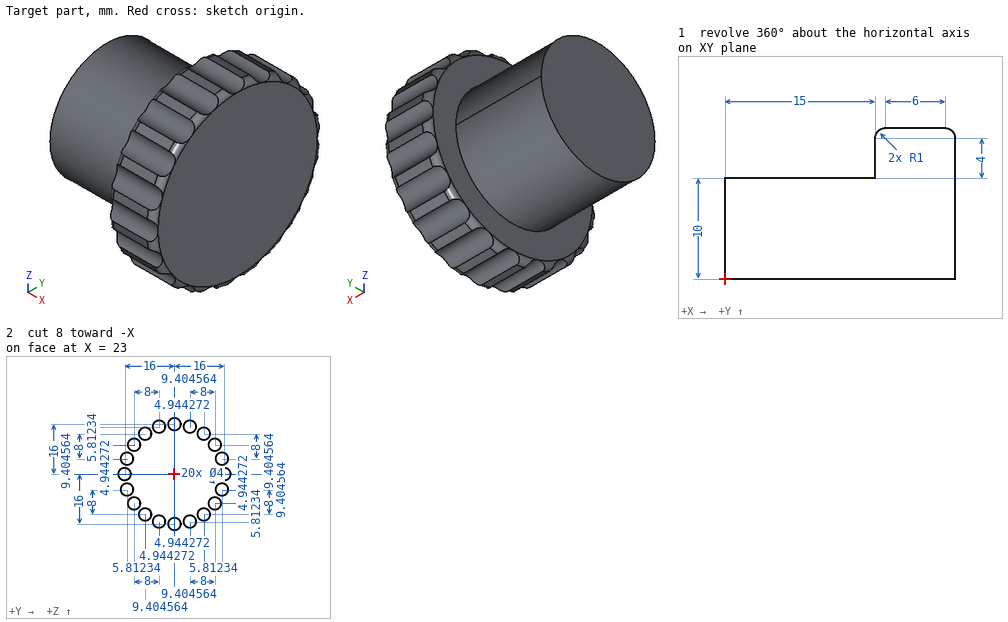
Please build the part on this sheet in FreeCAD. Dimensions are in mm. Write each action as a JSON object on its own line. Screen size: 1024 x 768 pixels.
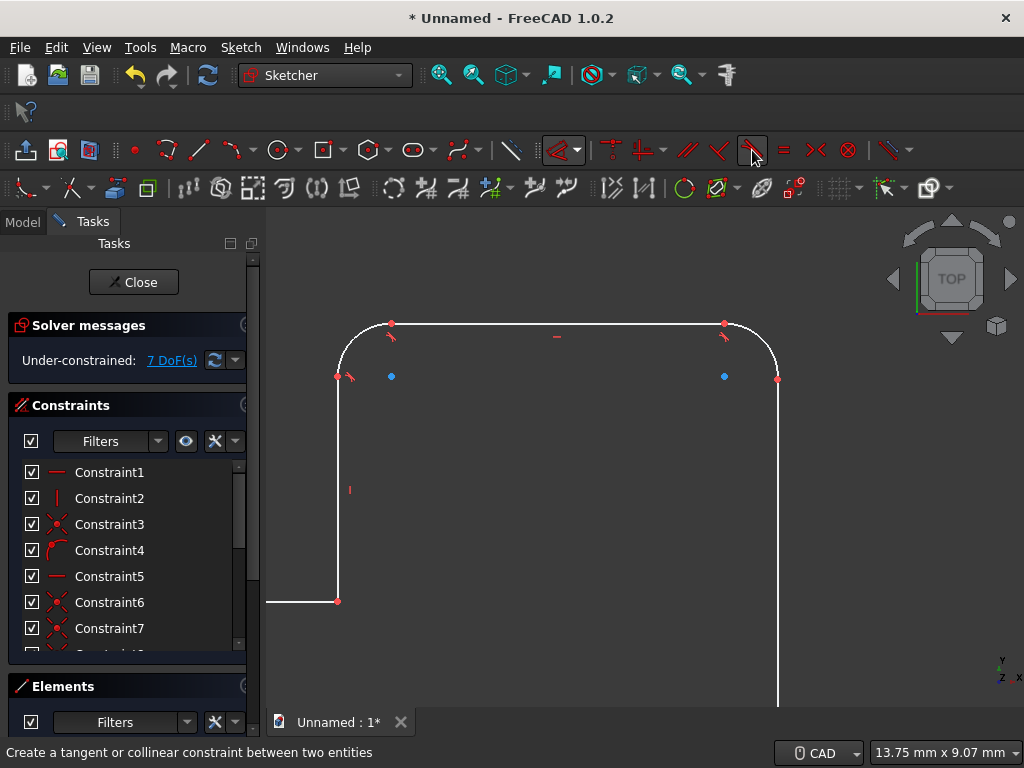
{"action": "left_click", "coordinate": [778, 611]}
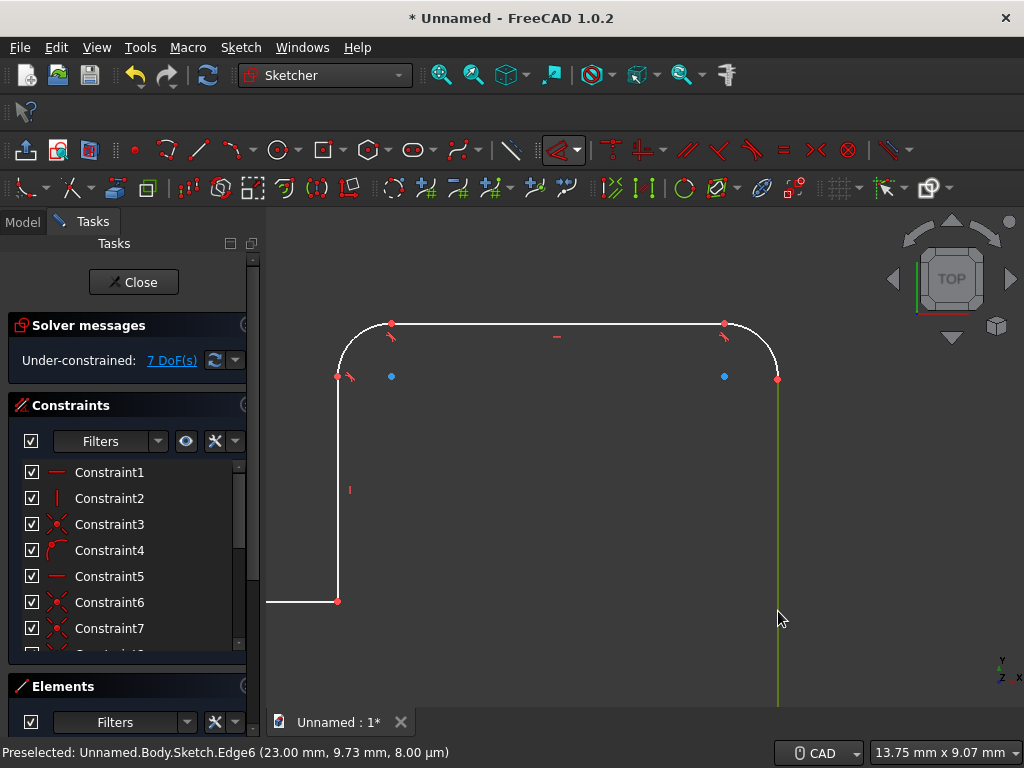
{"action": "left_click", "coordinate": [773, 355]}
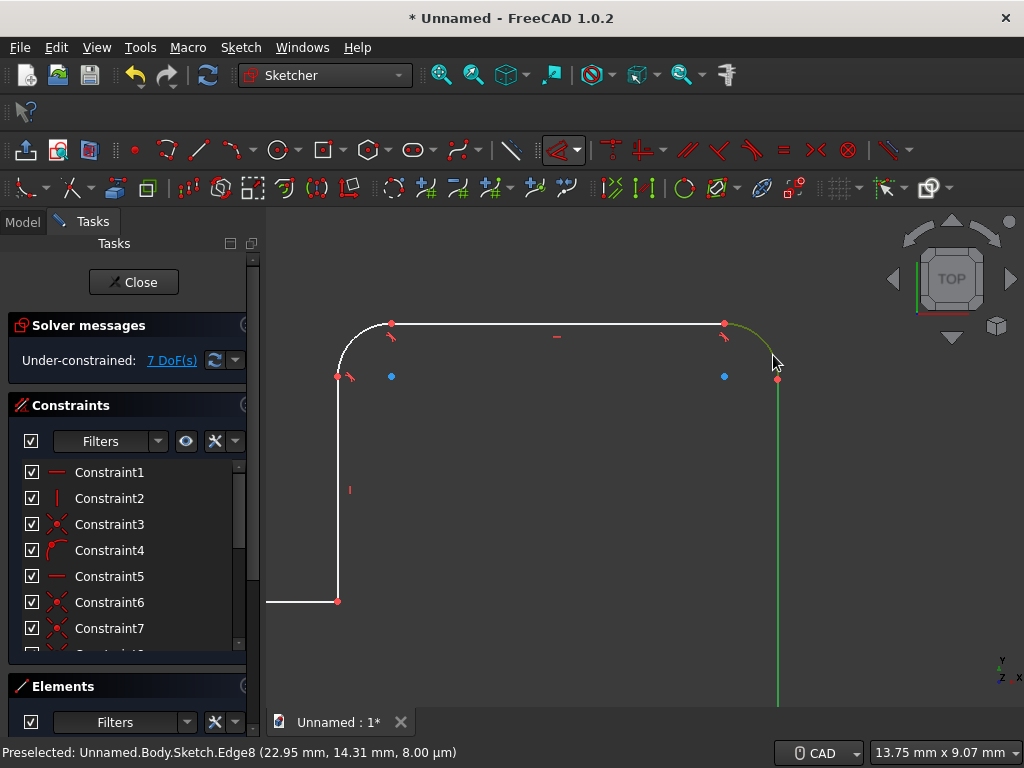
{"action": "left_click", "coordinate": [752, 150]}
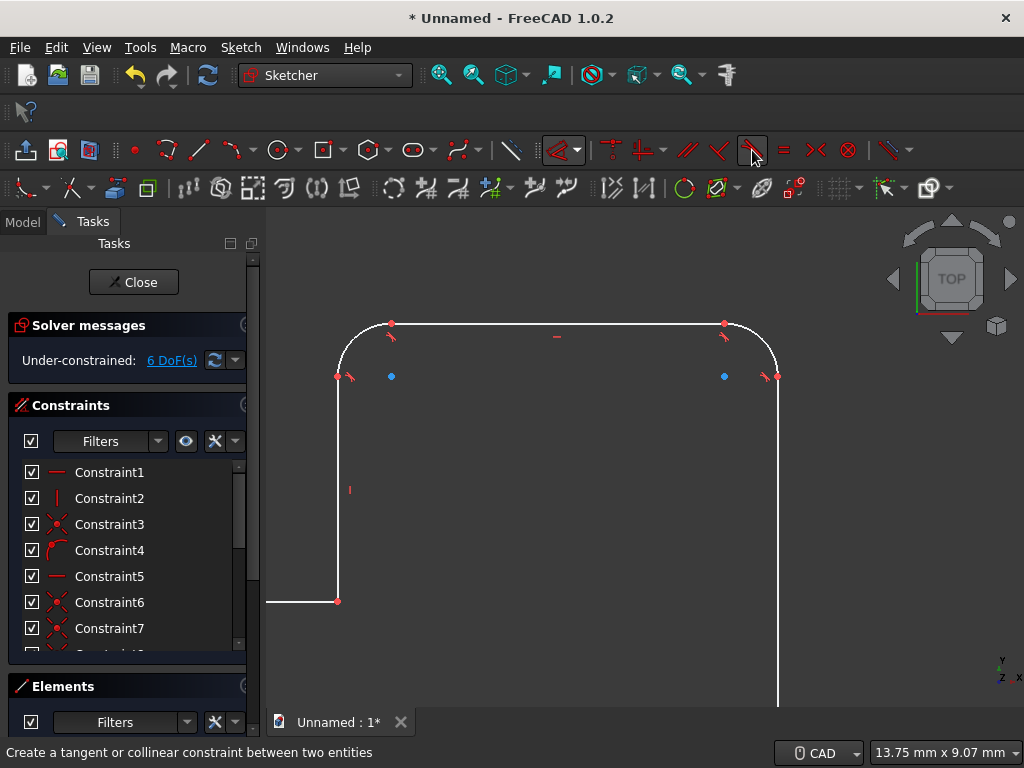
{"action": "left_click", "coordinate": [367, 329]}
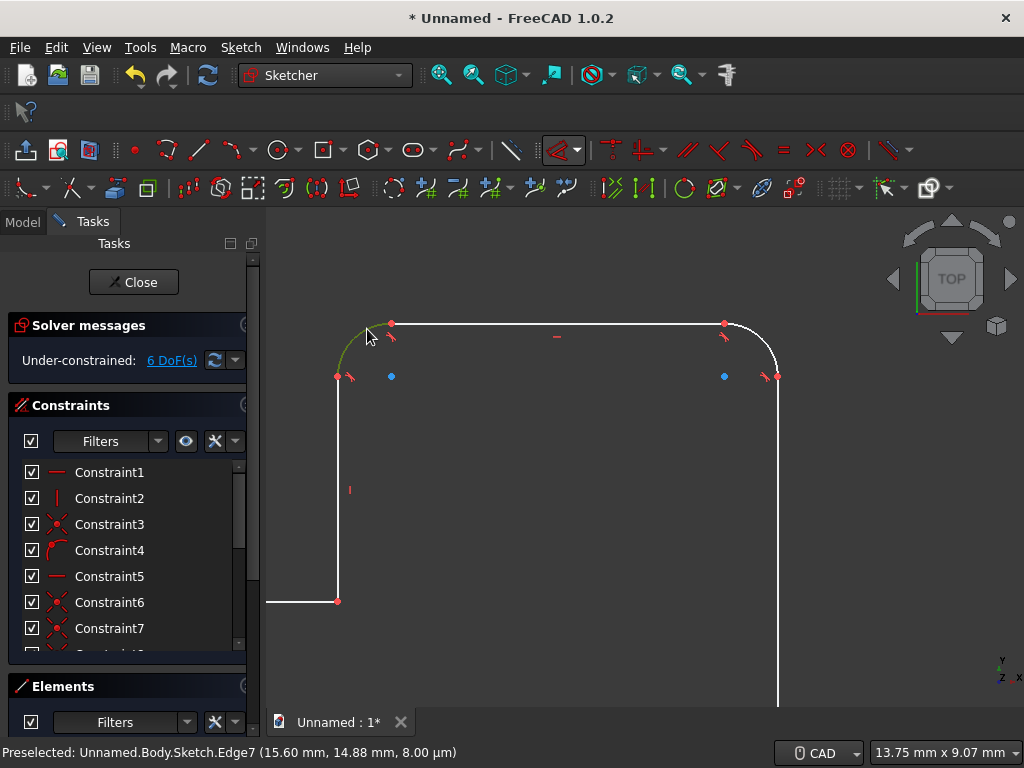
{"action": "left_click", "coordinate": [772, 353]}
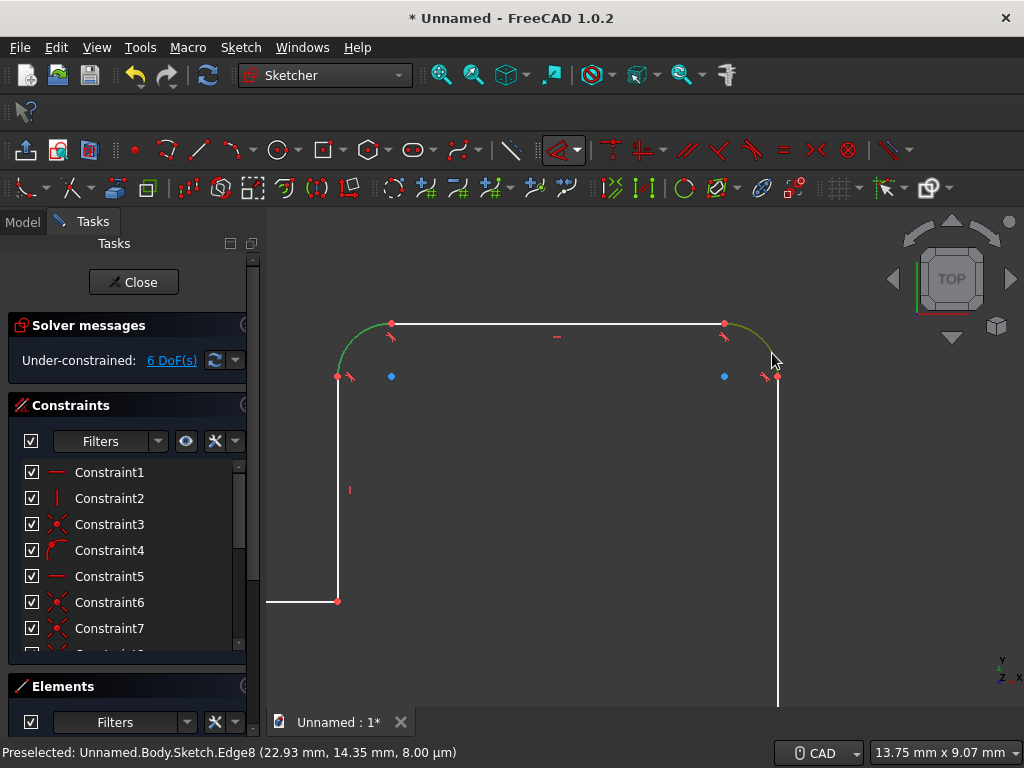
{"action": "left_click", "coordinate": [784, 150]}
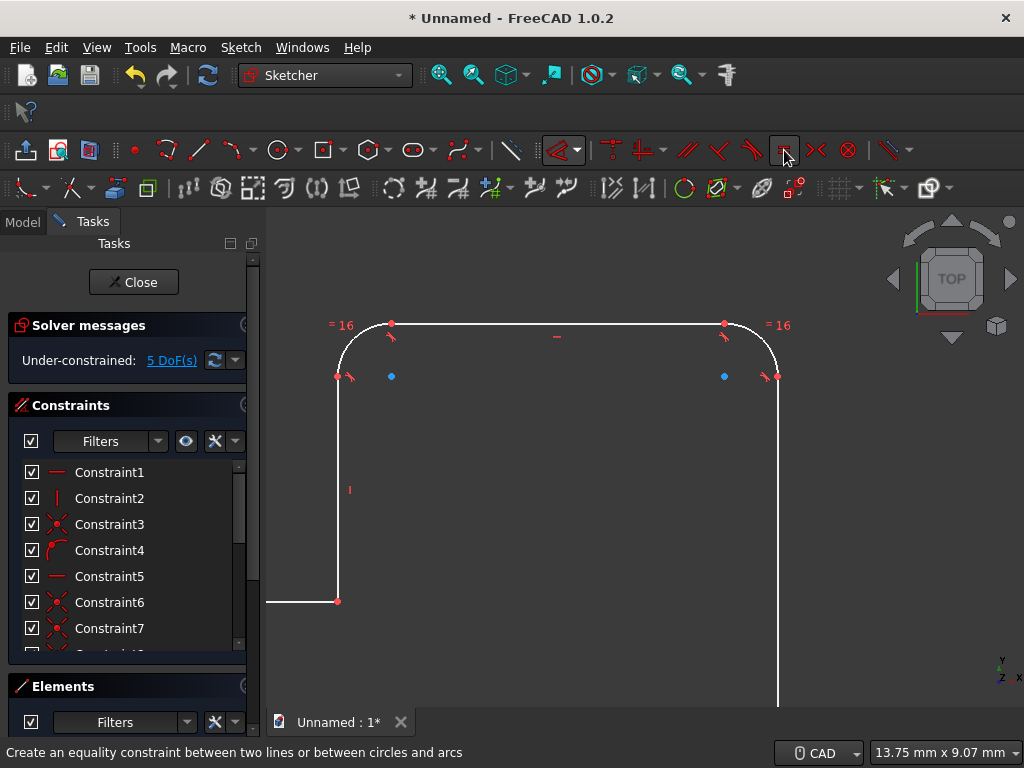
{"action": "left_click", "coordinate": [558, 150]}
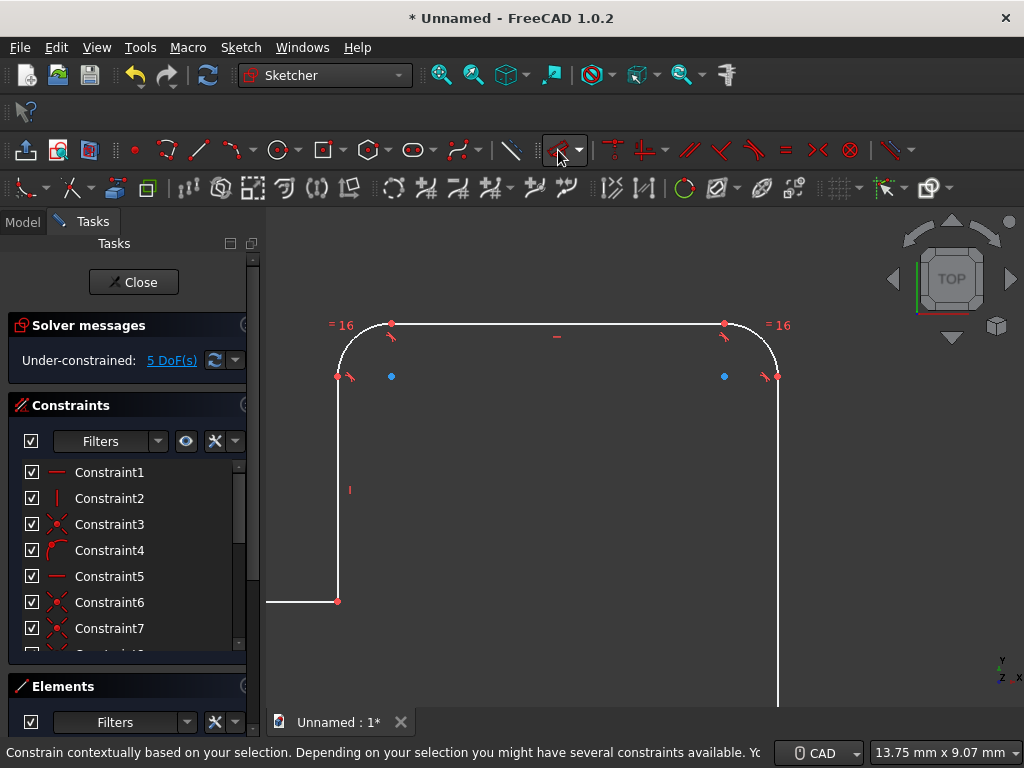
{"action": "left_click", "coordinate": [367, 329]}
{"action": "left_click", "coordinate": [353, 300]}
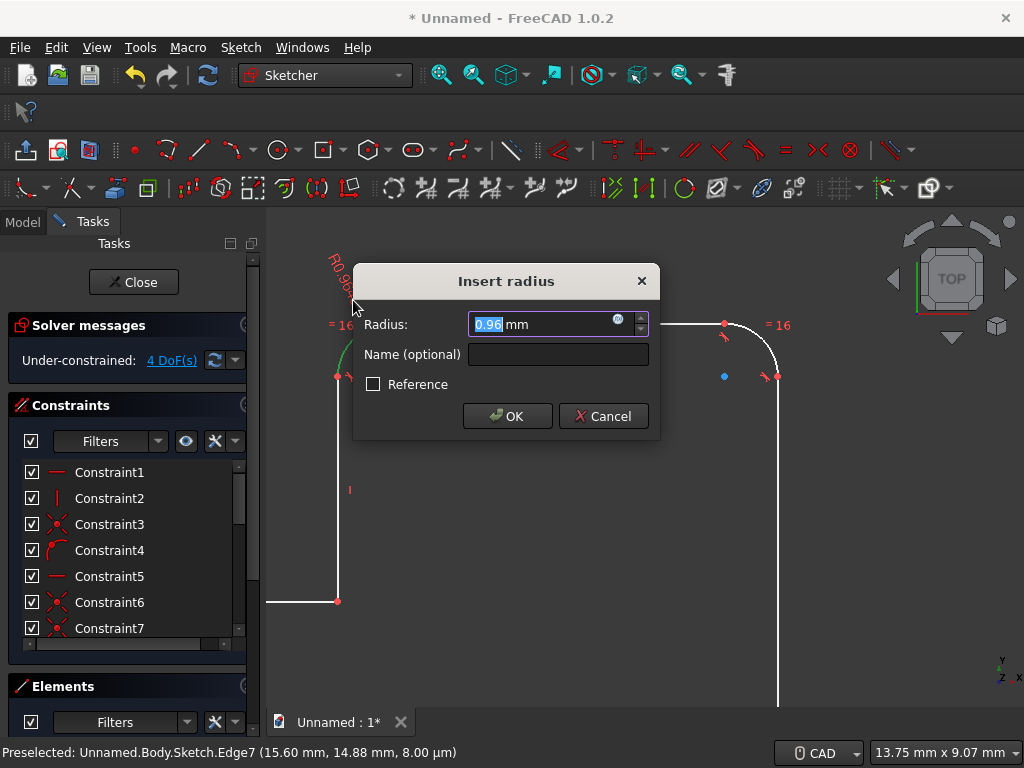
{"action": "type", "text": "1"}
{"action": "key", "text": "Return"}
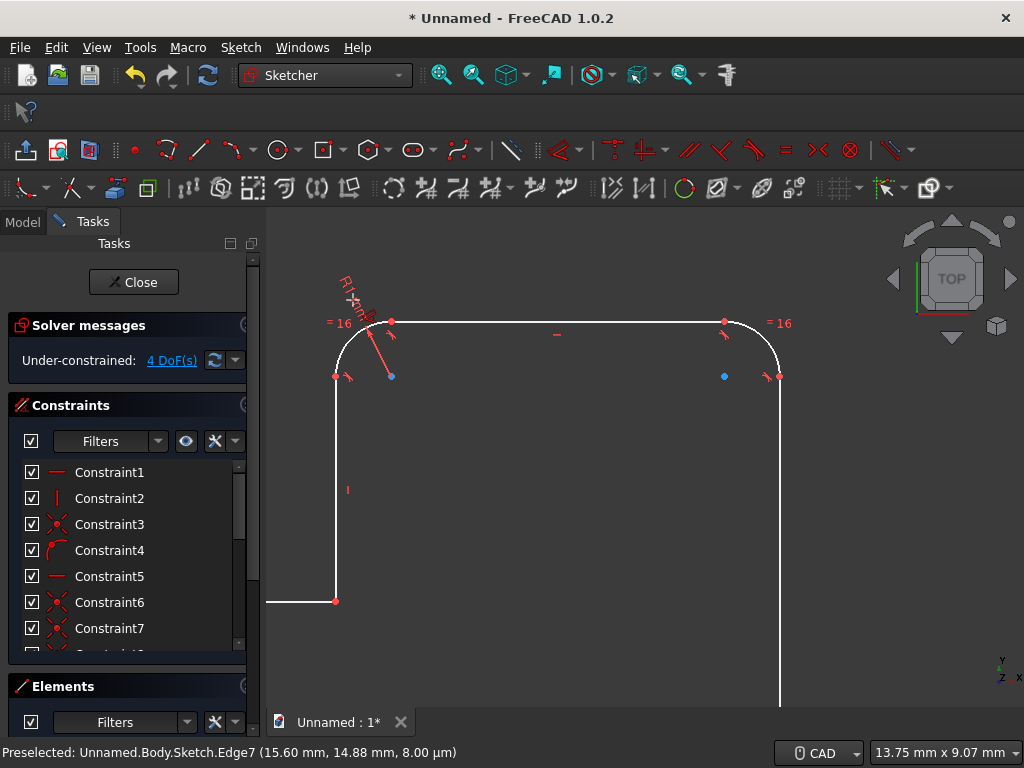
{"action": "left_click", "coordinate": [625, 322]}
{"action": "left_click", "coordinate": [558, 288]}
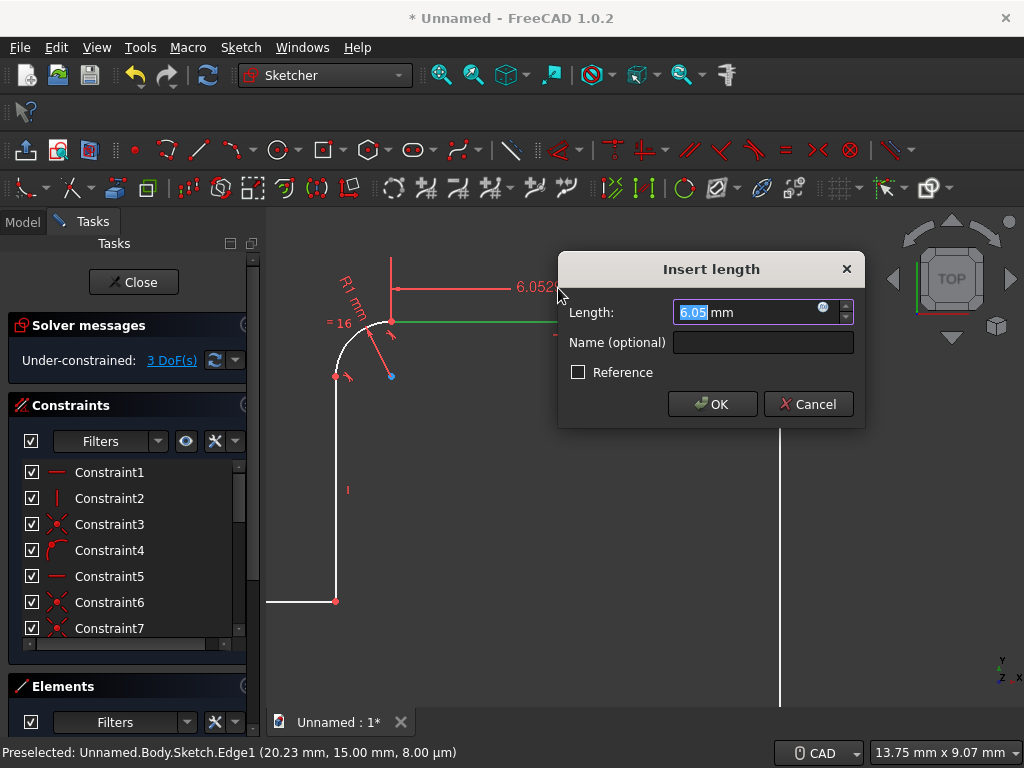
{"action": "type", "text": "6"}
{"action": "key", "text": "Return"}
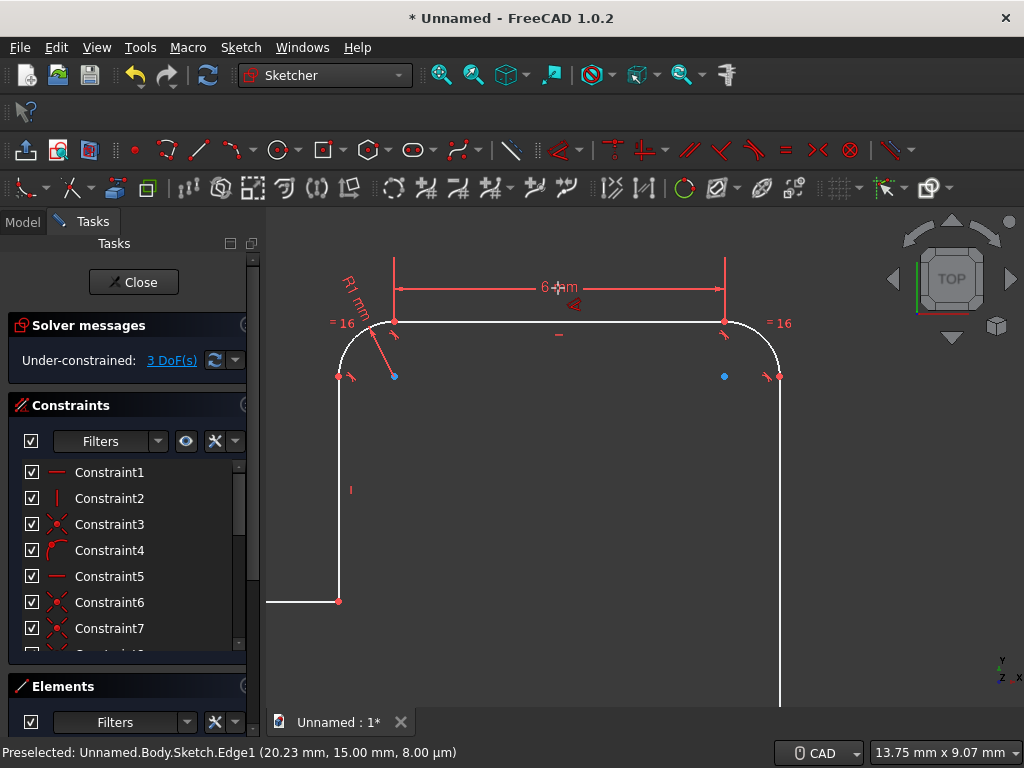
{"action": "left_click", "coordinate": [339, 444]}
{"action": "left_click", "coordinate": [373, 489]}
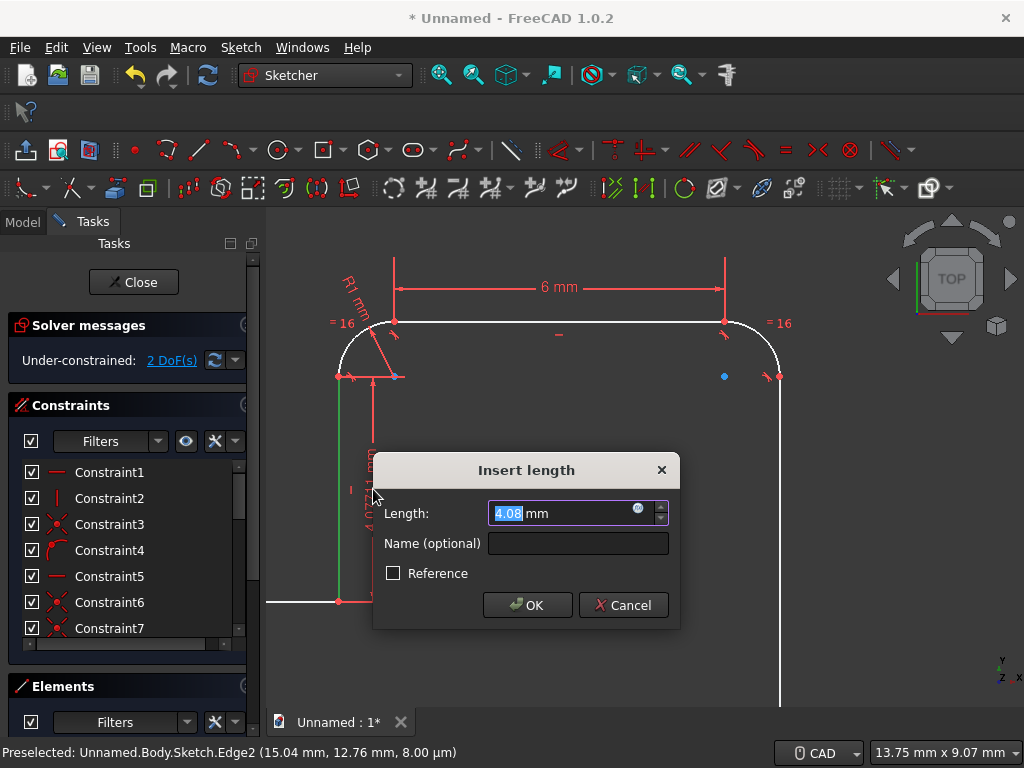
{"action": "type", "text": "4"}
{"action": "key", "text": "Return"}